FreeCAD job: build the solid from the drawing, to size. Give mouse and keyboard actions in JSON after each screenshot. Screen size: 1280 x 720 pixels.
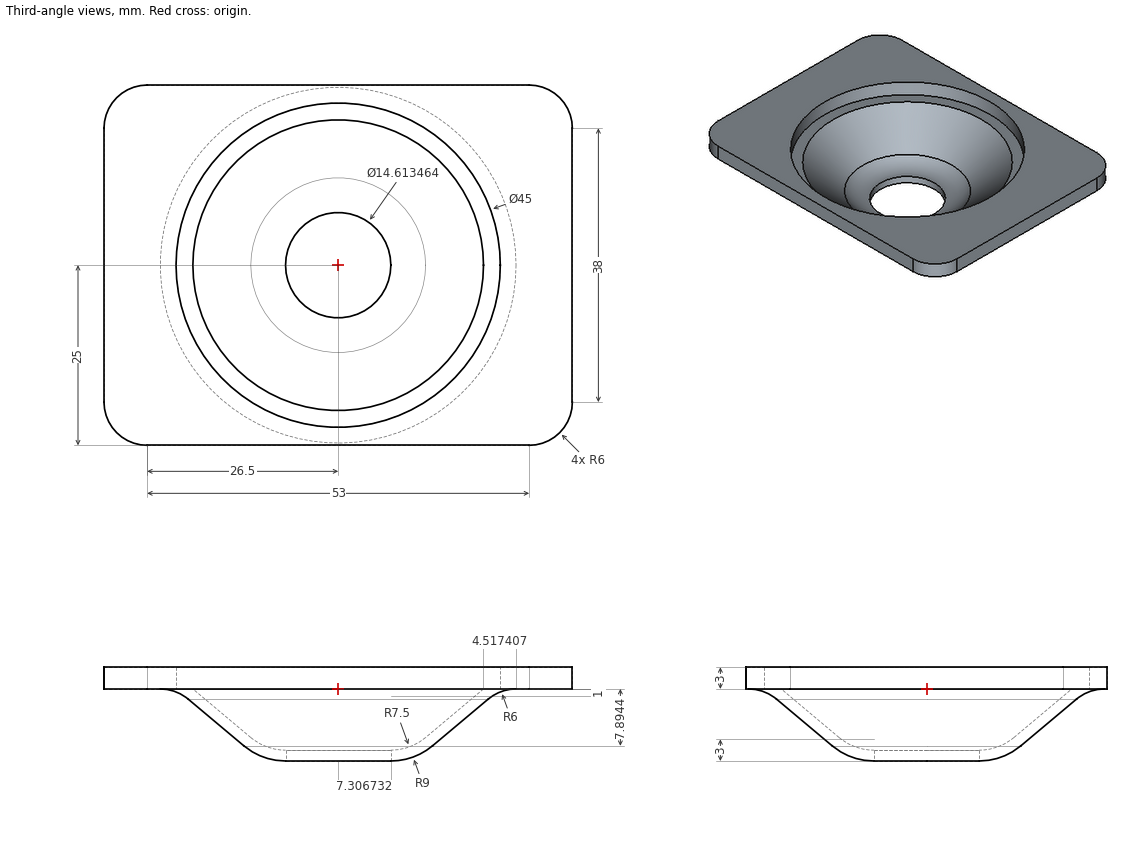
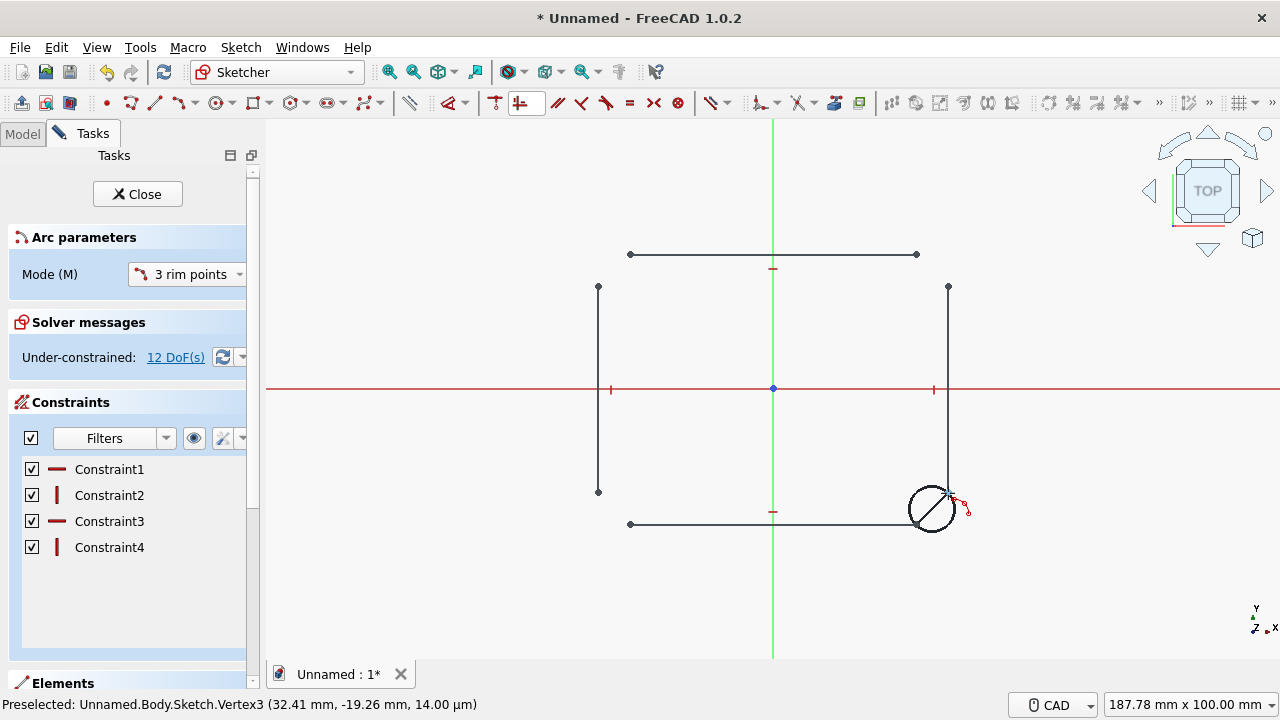
{"action": "scroll", "coordinate": [939, 515], "scroll_direction": "up", "scroll_amount": 3}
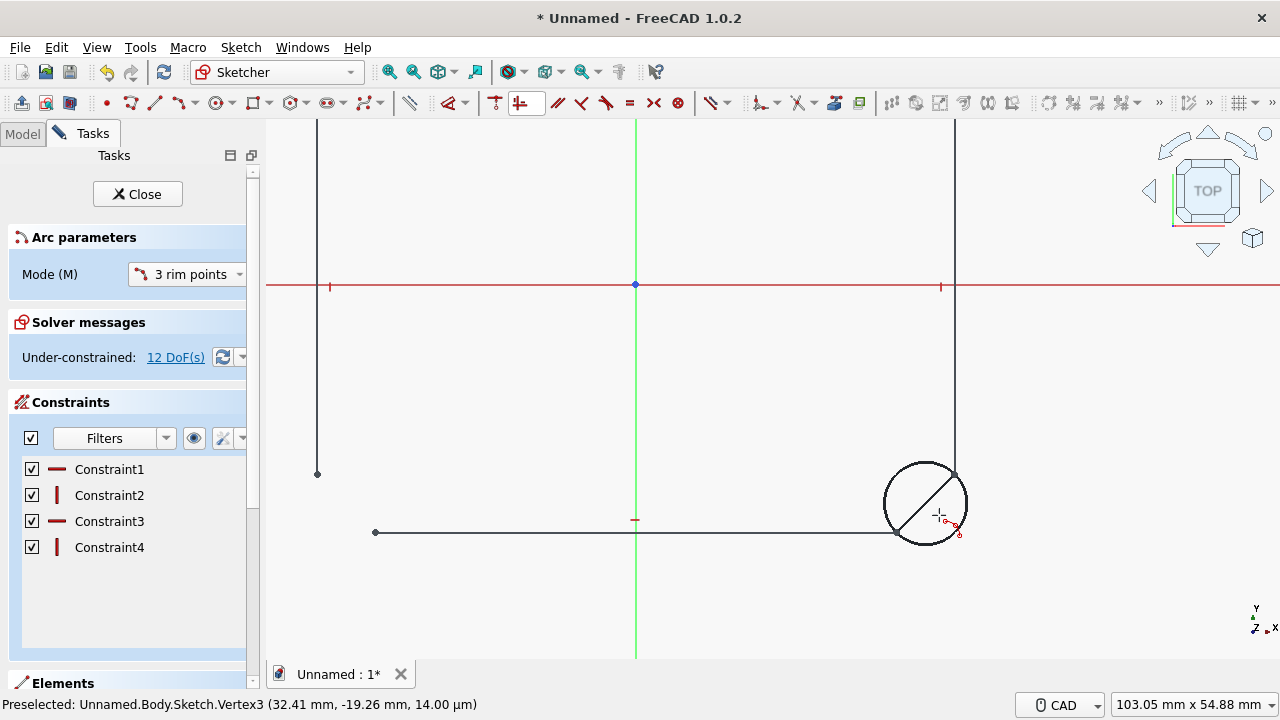
{"action": "left_click", "coordinate": [938, 514]}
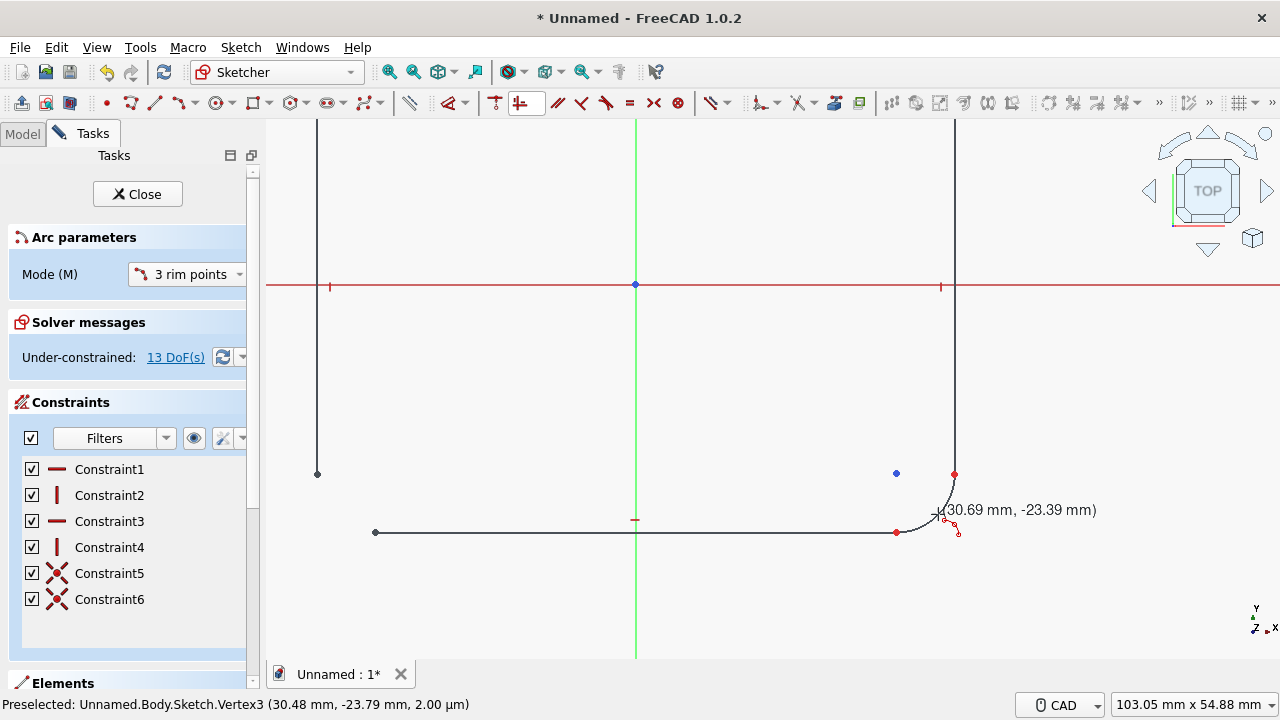
{"action": "scroll", "coordinate": [844, 601], "scroll_direction": "down", "scroll_amount": 2}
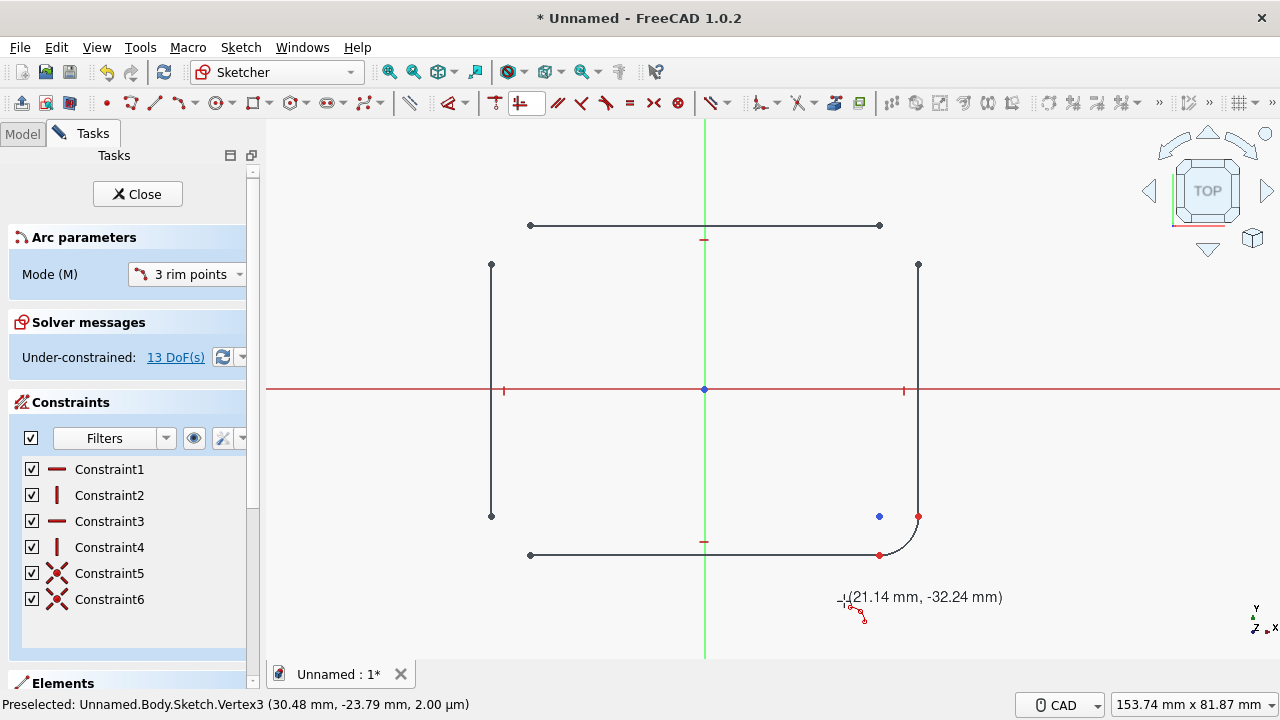
{"action": "left_click", "coordinate": [918, 265]}
{"action": "left_click", "coordinate": [879, 226]}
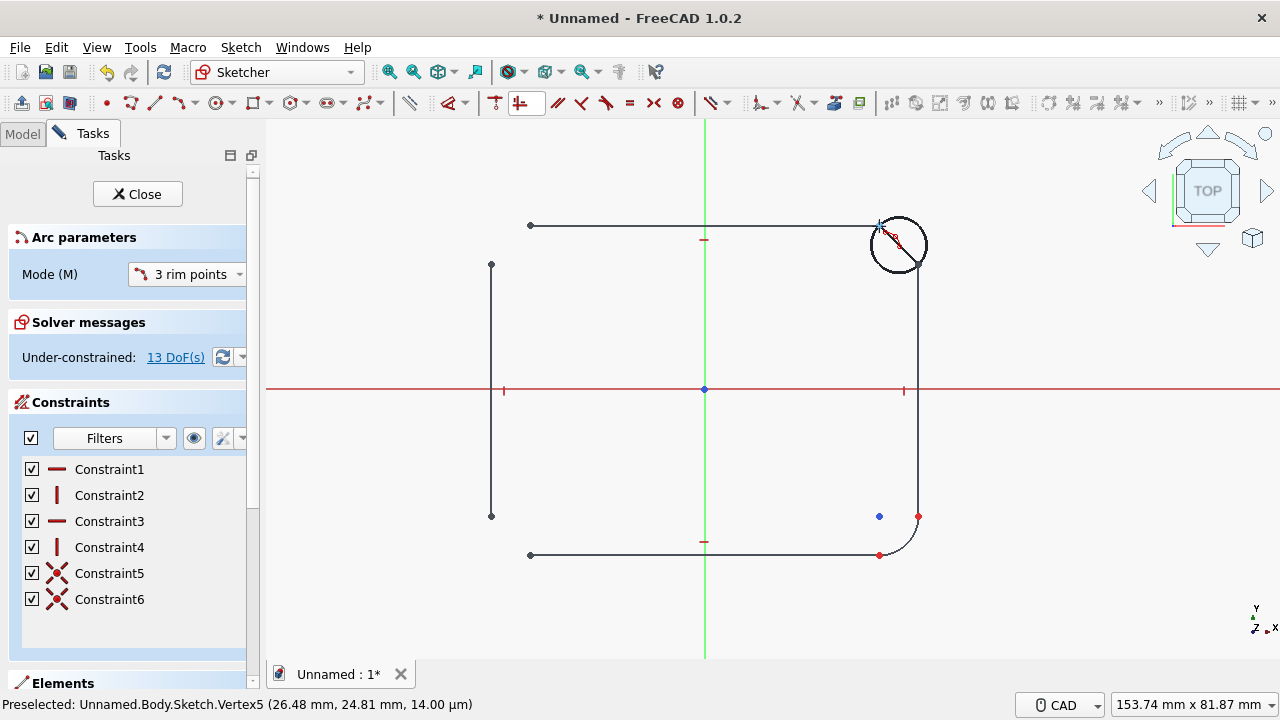
{"action": "scroll", "coordinate": [908, 236], "scroll_direction": "up", "scroll_amount": 2}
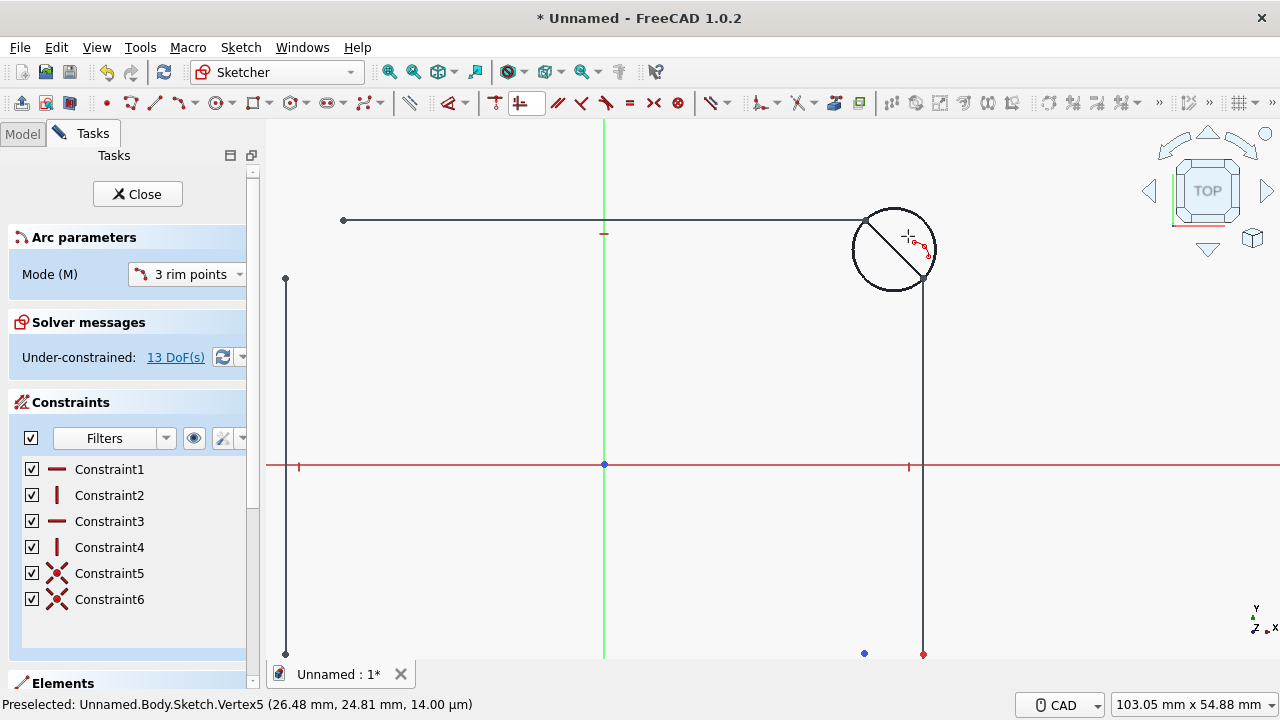
{"action": "left_click", "coordinate": [907, 236]}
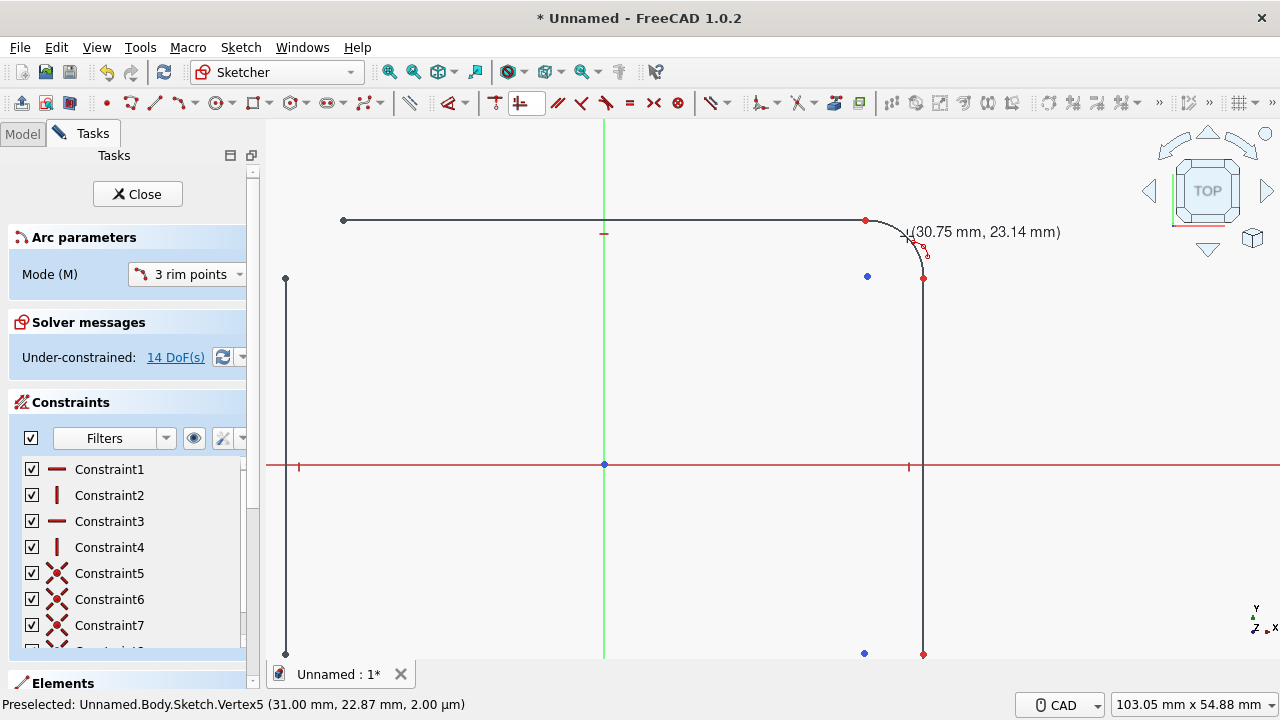
{"action": "left_click", "coordinate": [344, 220]}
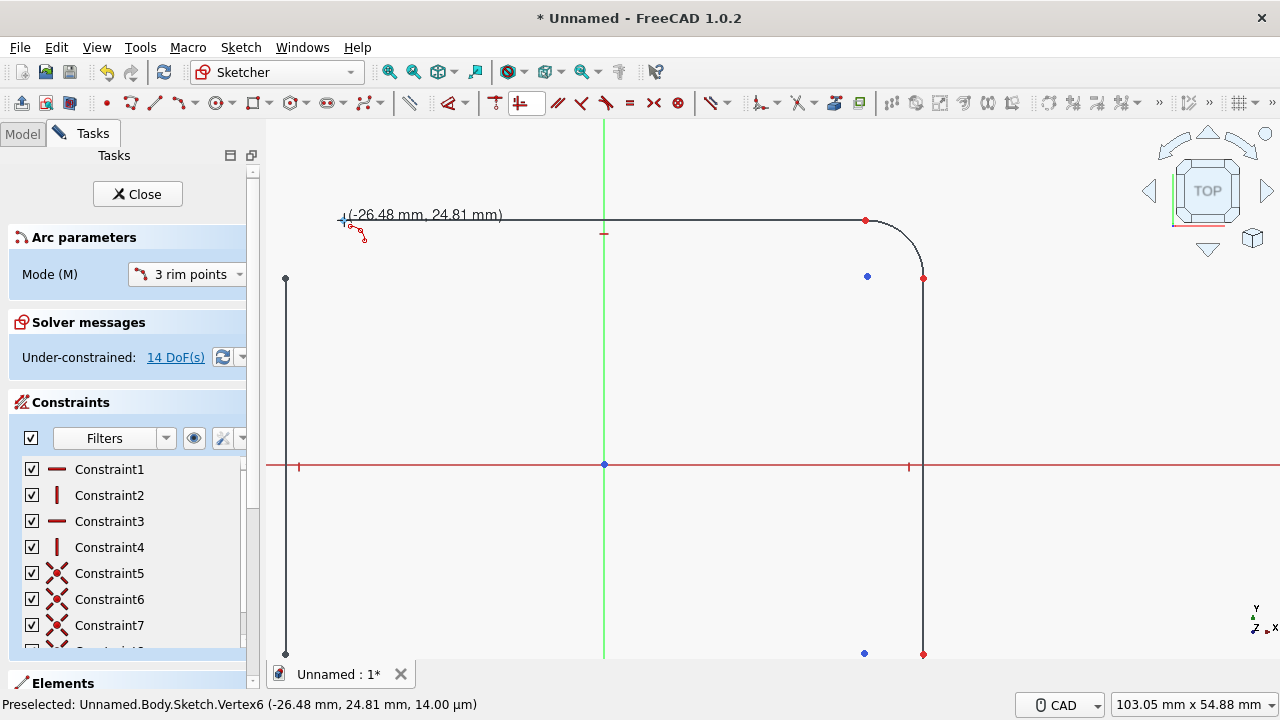
{"action": "scroll", "coordinate": [908, 235], "scroll_direction": "down", "scroll_amount": 2}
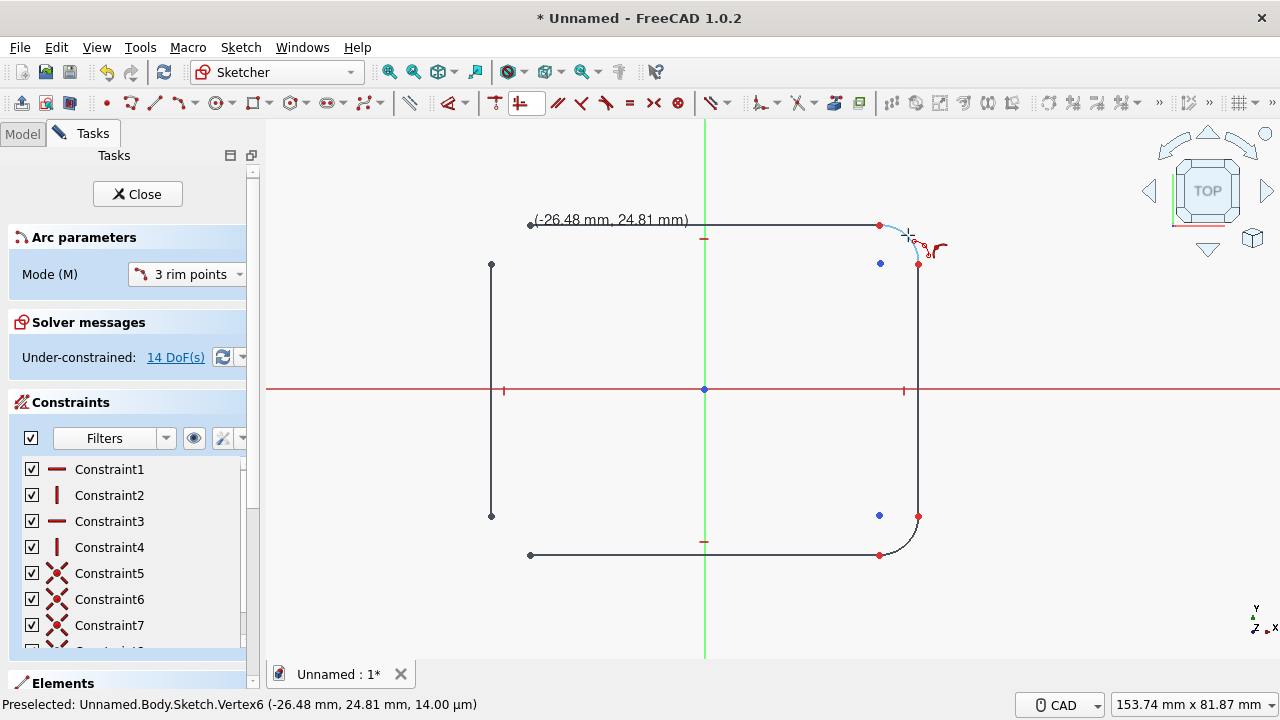
{"action": "left_click", "coordinate": [491, 264]}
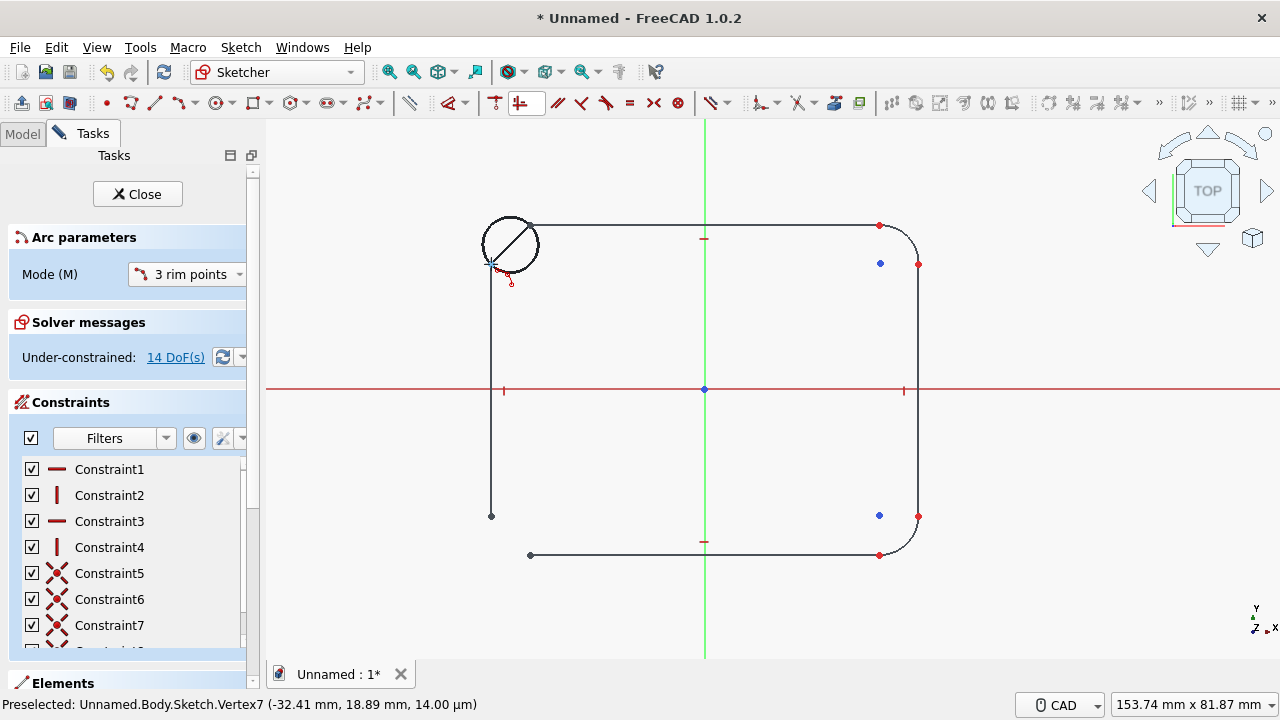
{"action": "scroll", "coordinate": [502, 236], "scroll_direction": "up", "scroll_amount": 2}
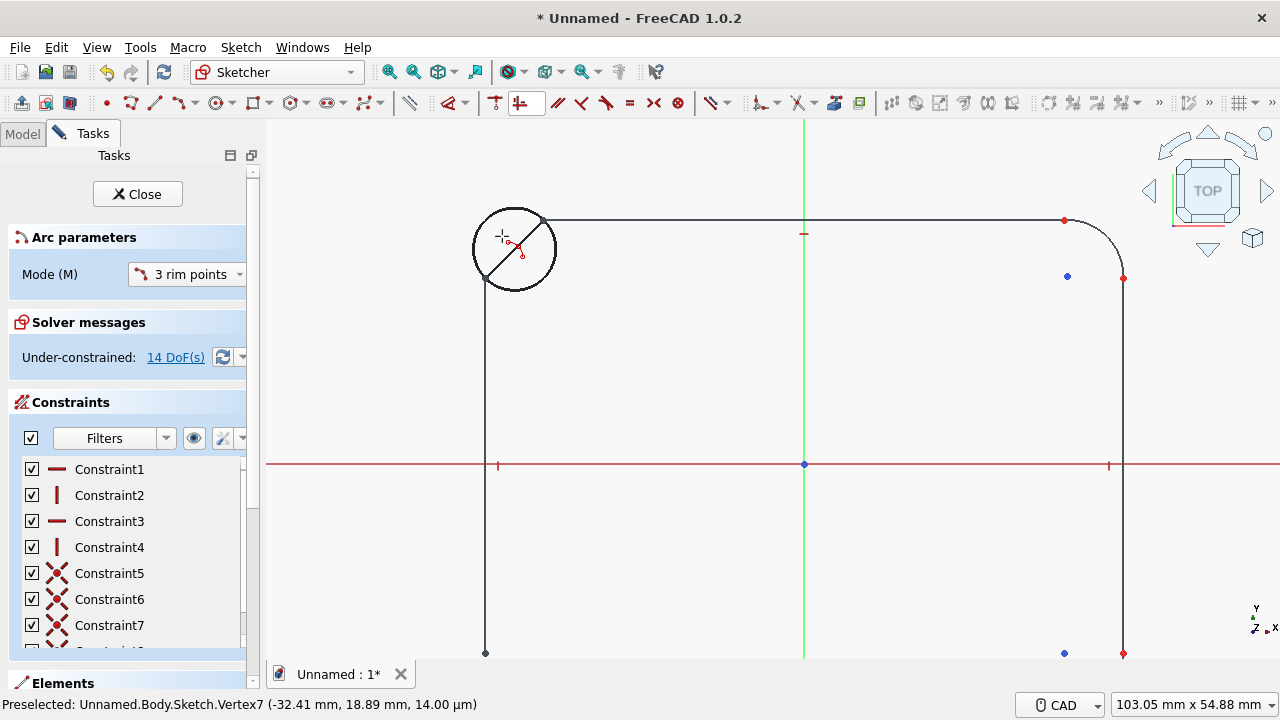
{"action": "left_click", "coordinate": [502, 235]}